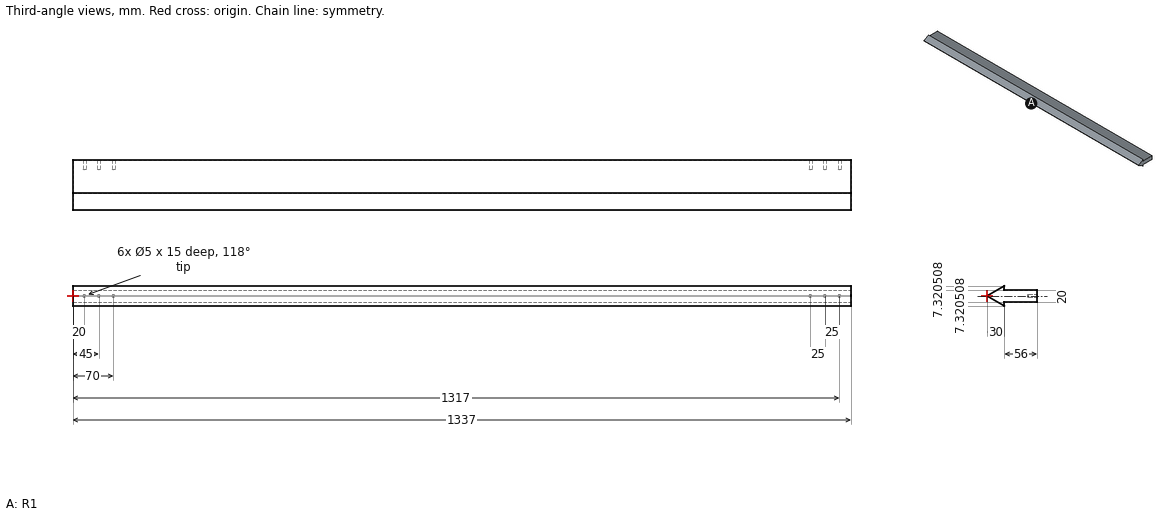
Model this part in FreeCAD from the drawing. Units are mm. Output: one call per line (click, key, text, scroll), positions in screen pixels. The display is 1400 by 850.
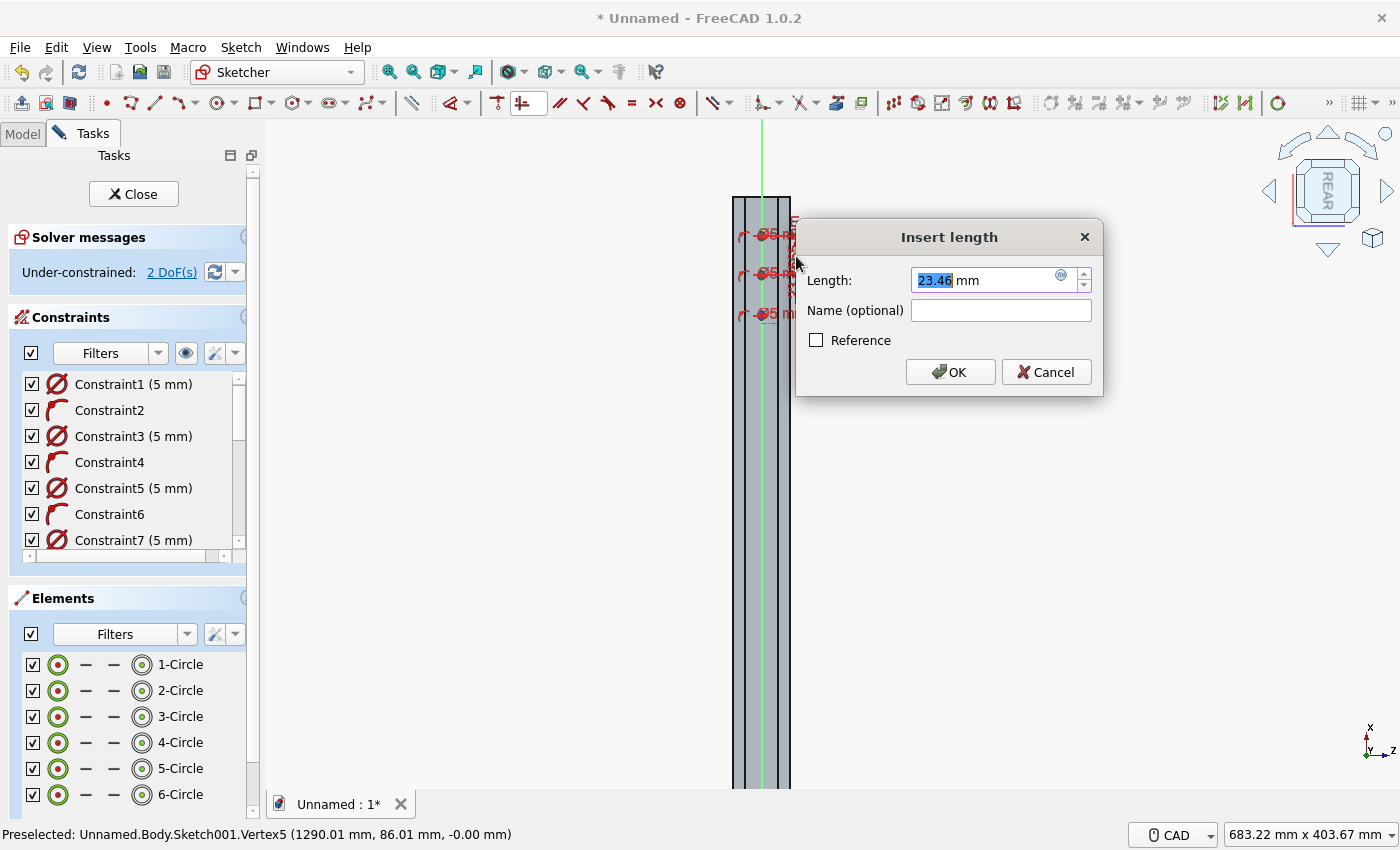
text(25)
key(Return)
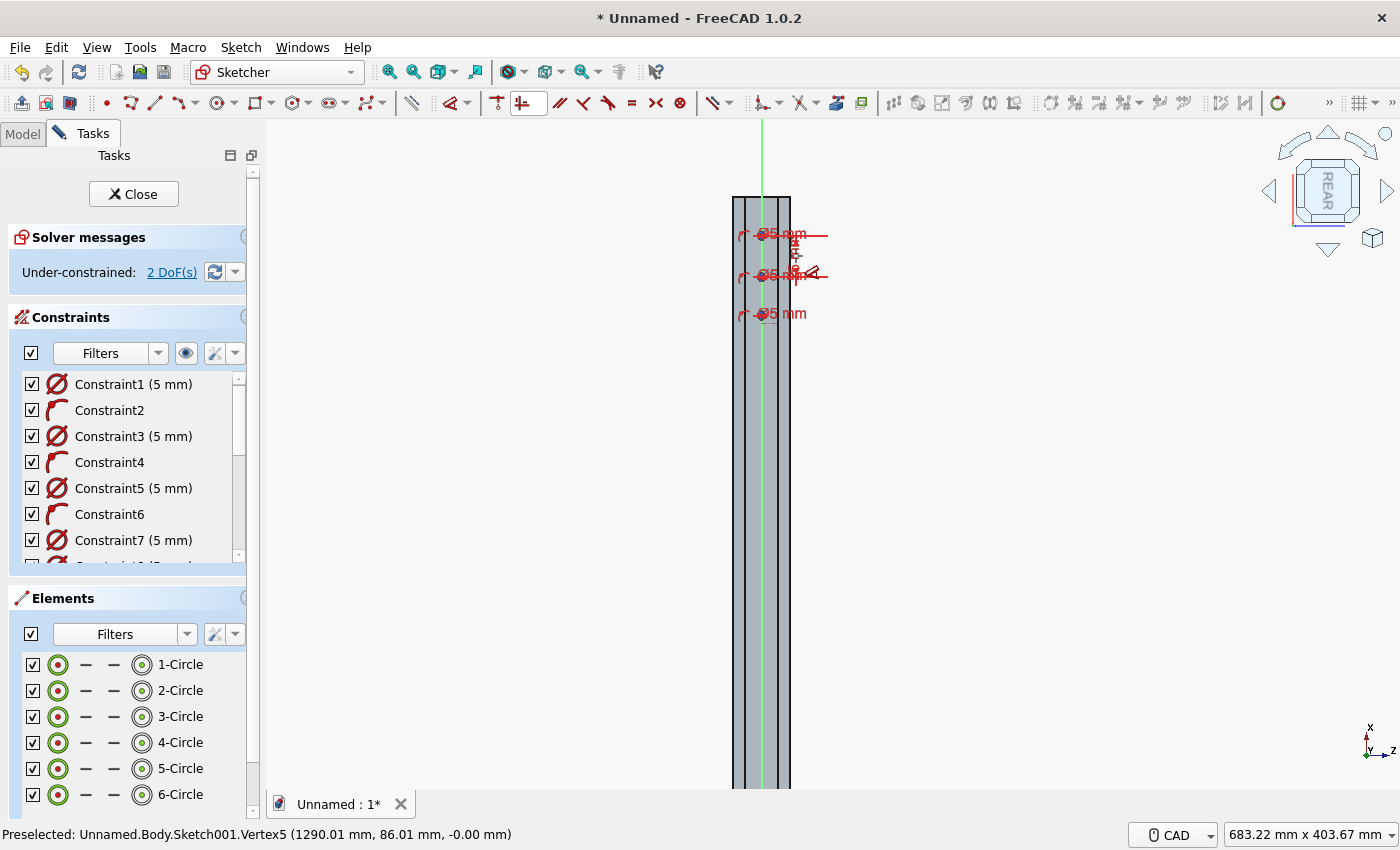
click(762, 277)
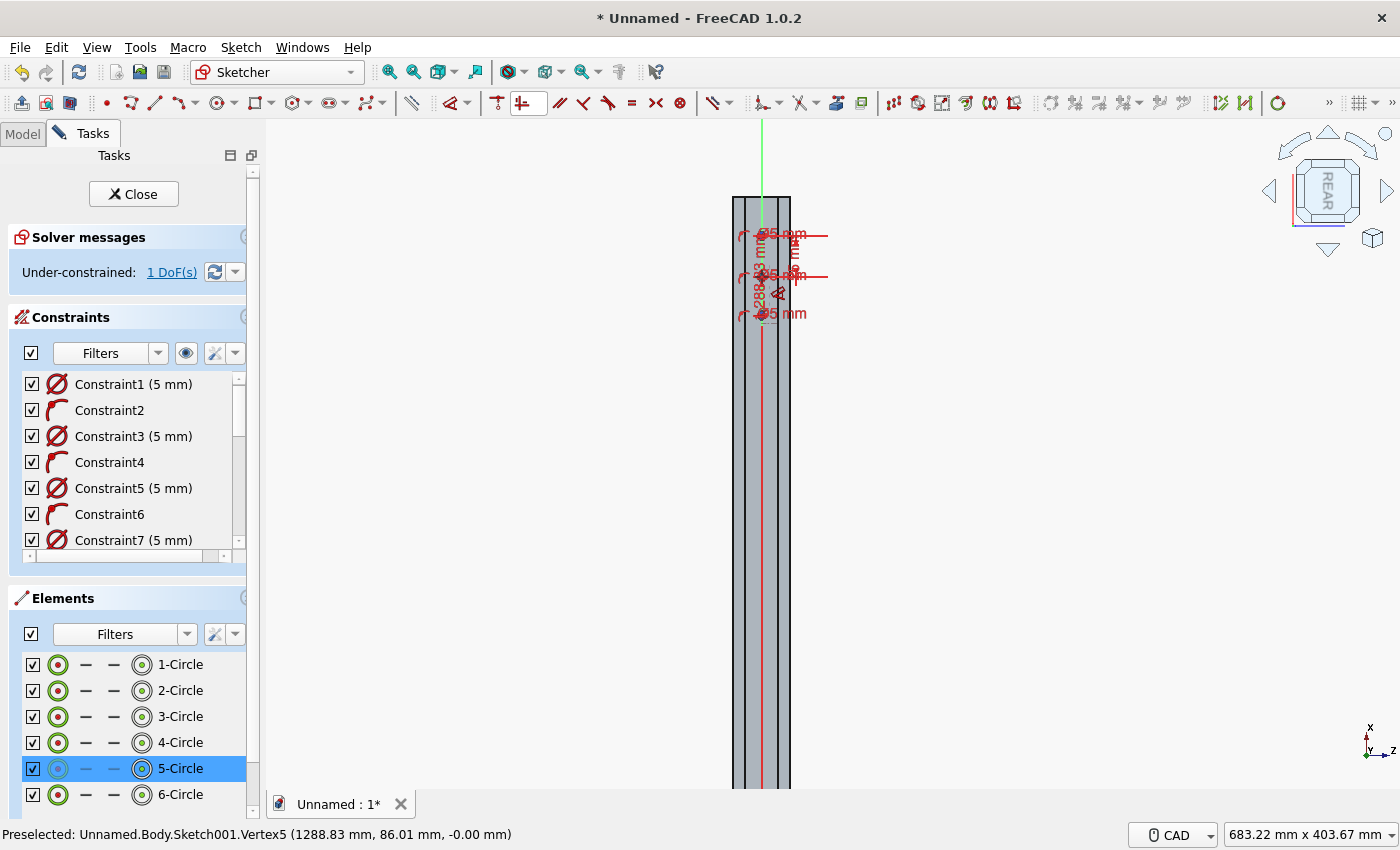
click(762, 316)
click(796, 296)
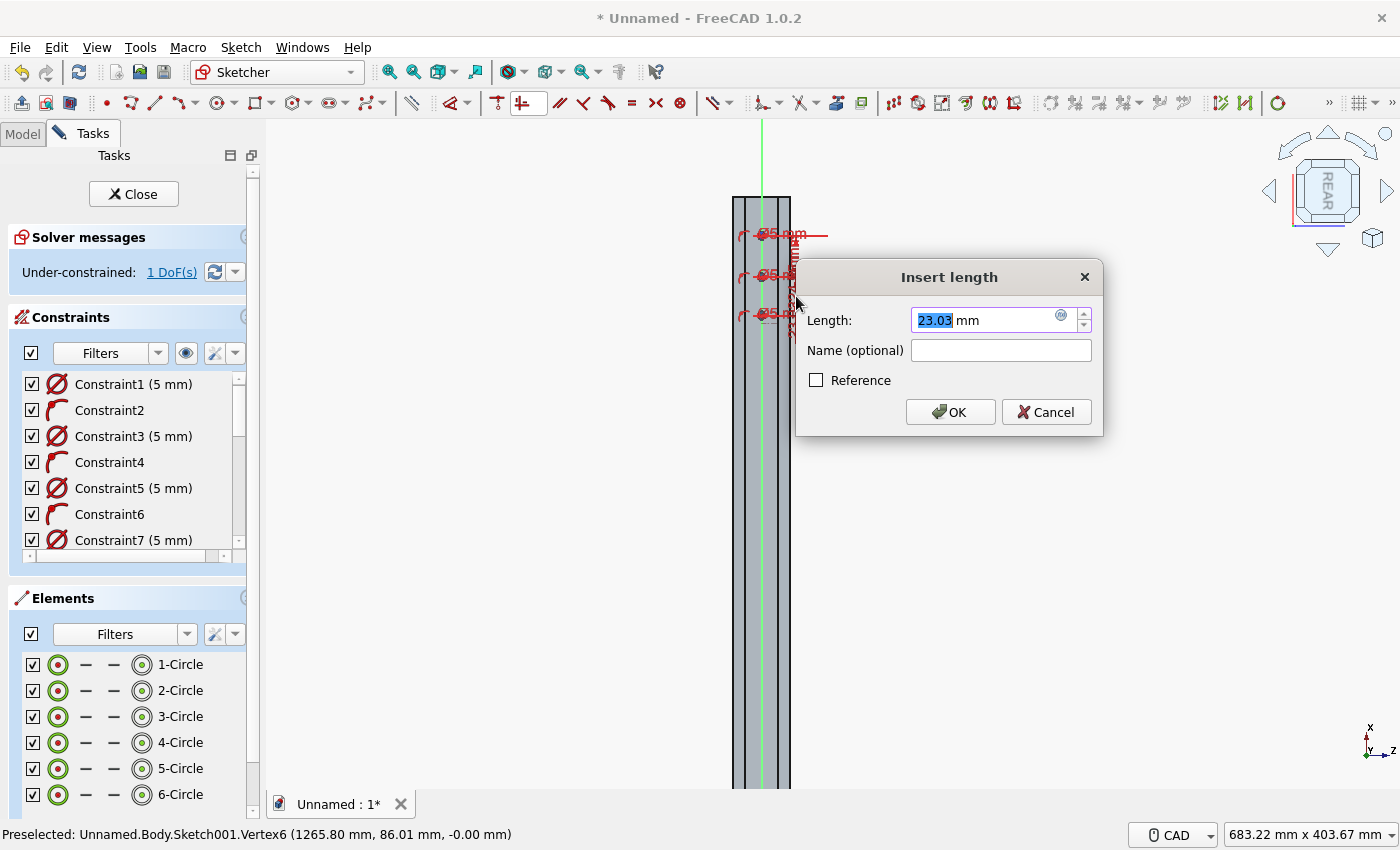
text(25)
key(Return)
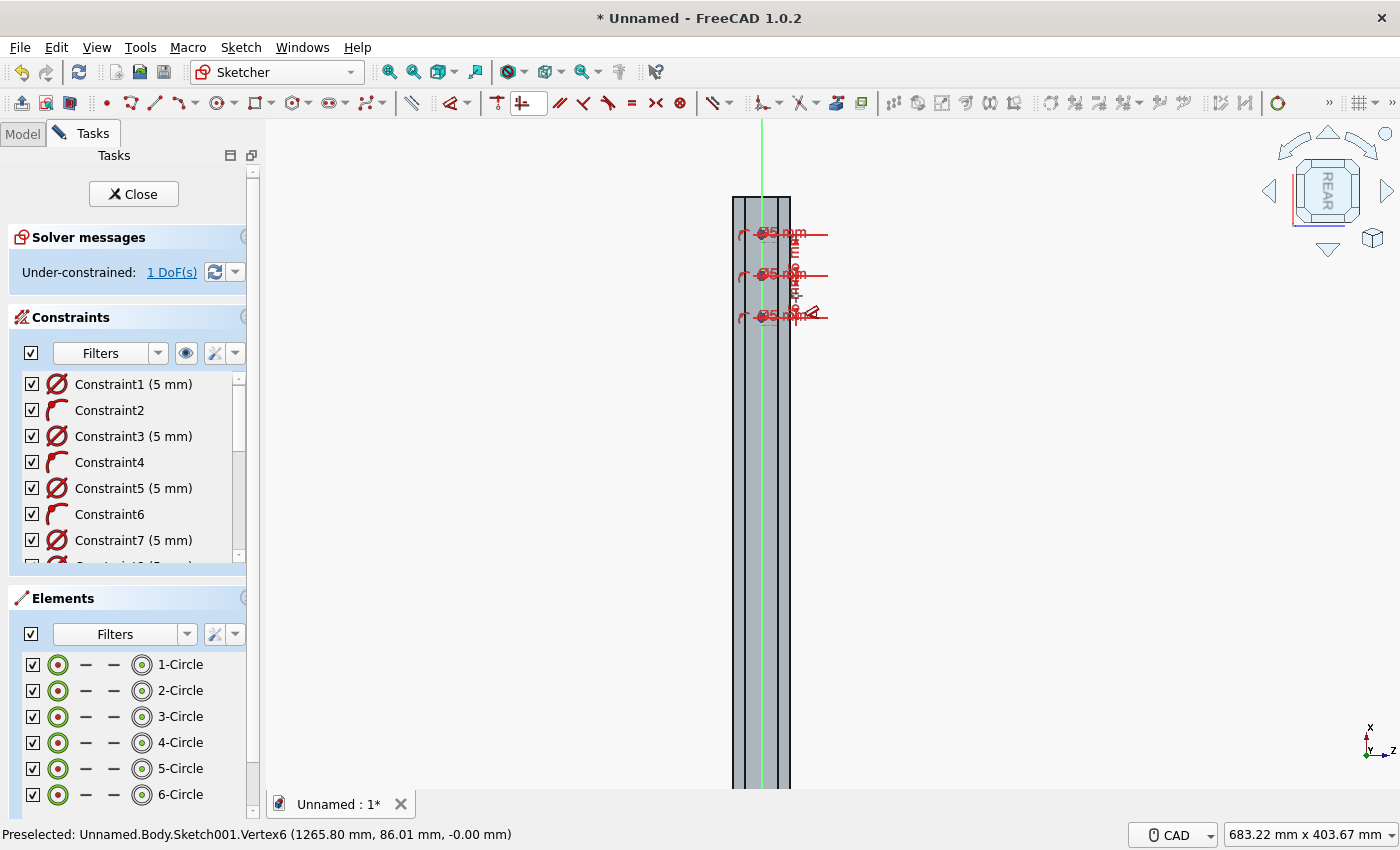
scroll(765, 235, down, 8)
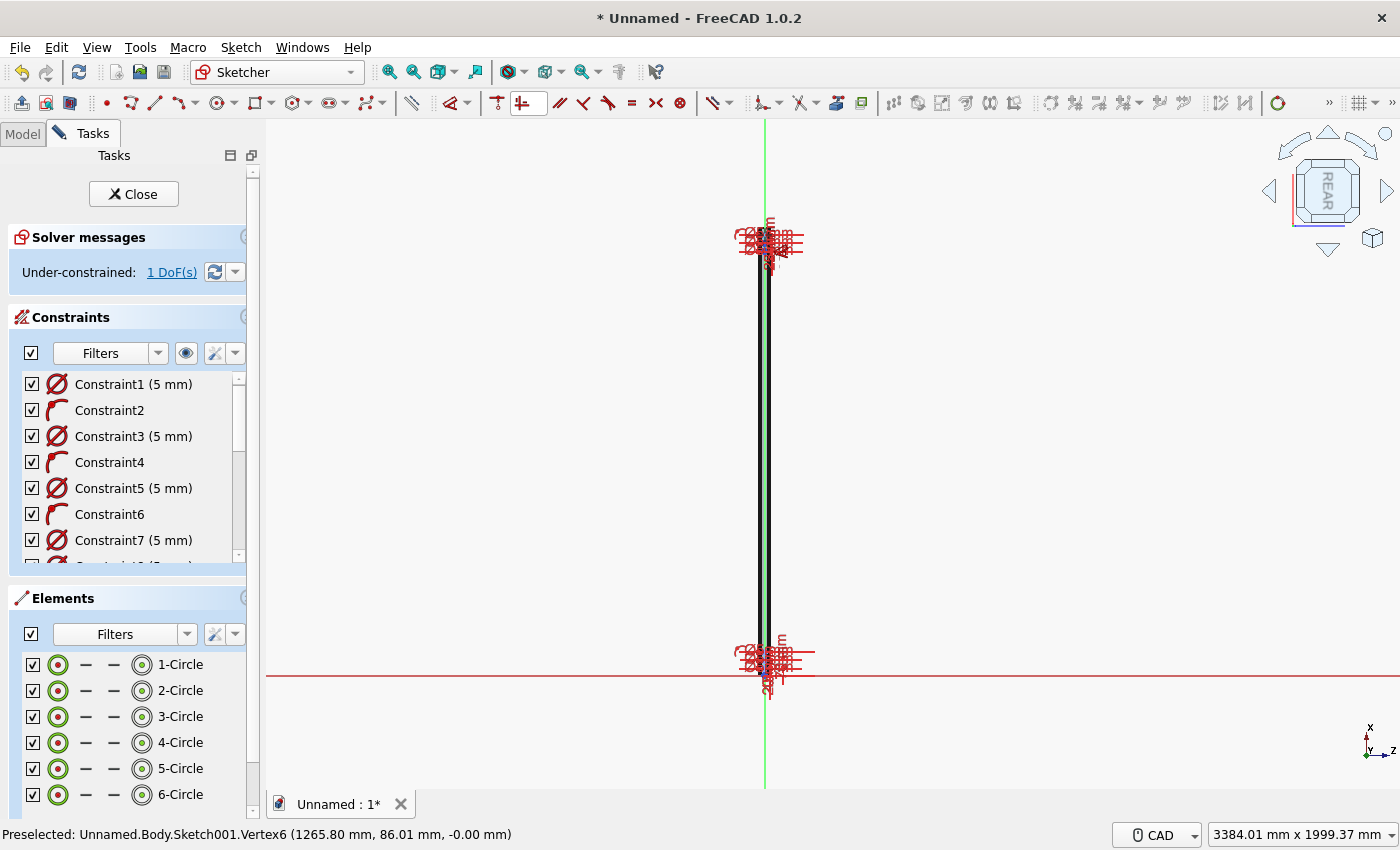
scroll(765, 235, up, 2)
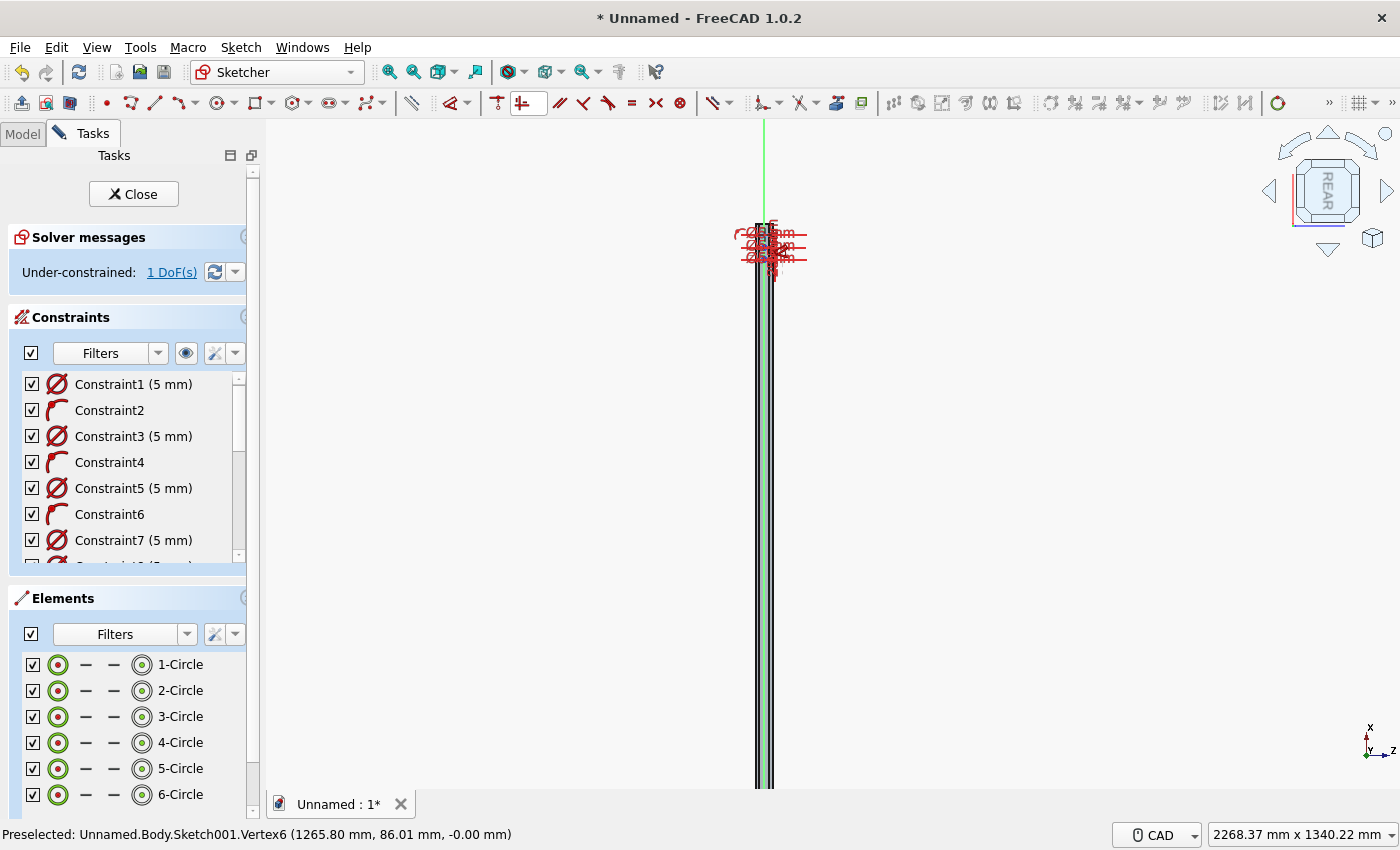
click(764, 235)
click(798, 498)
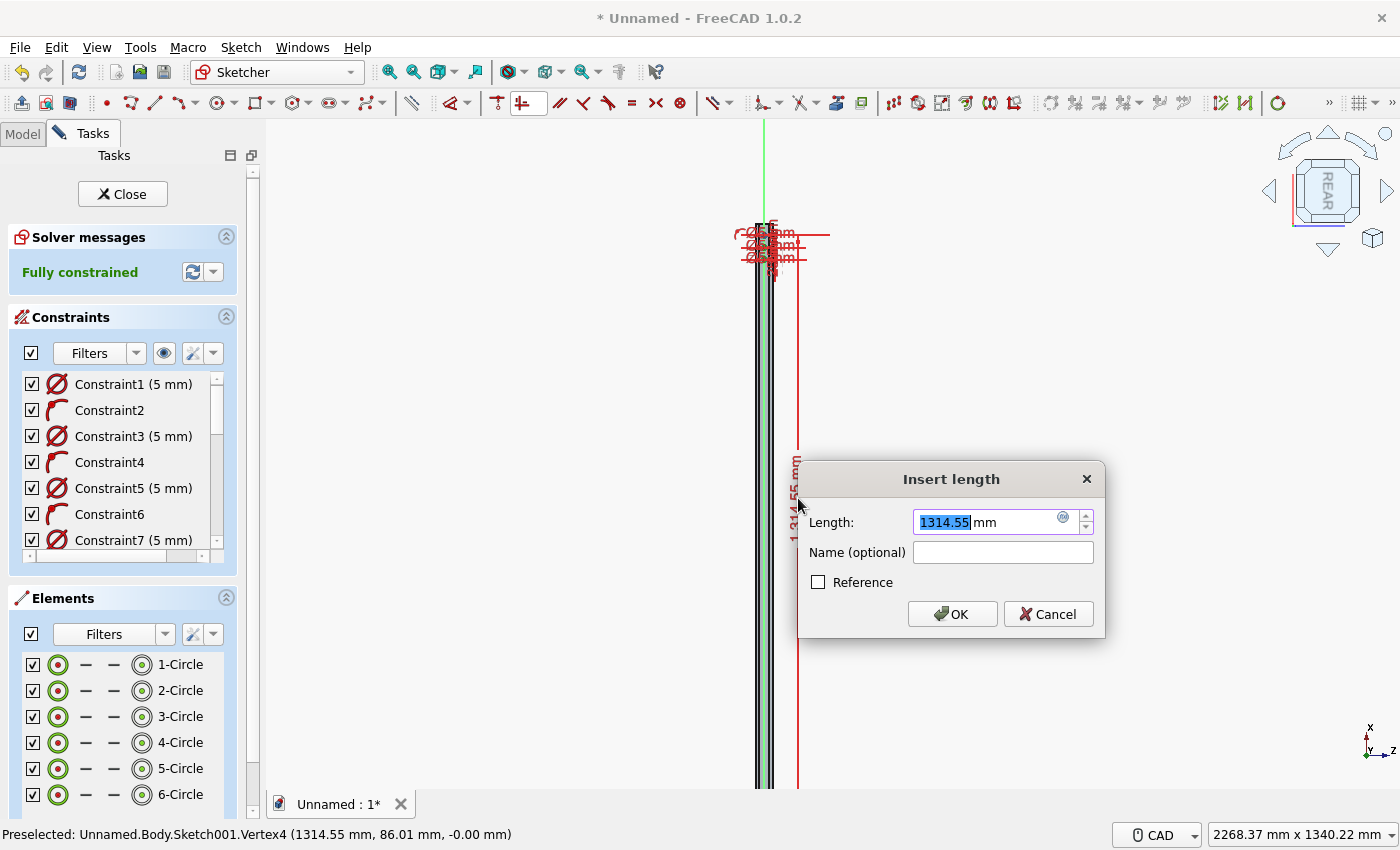
text(1317)
key(Return)
key(Escape)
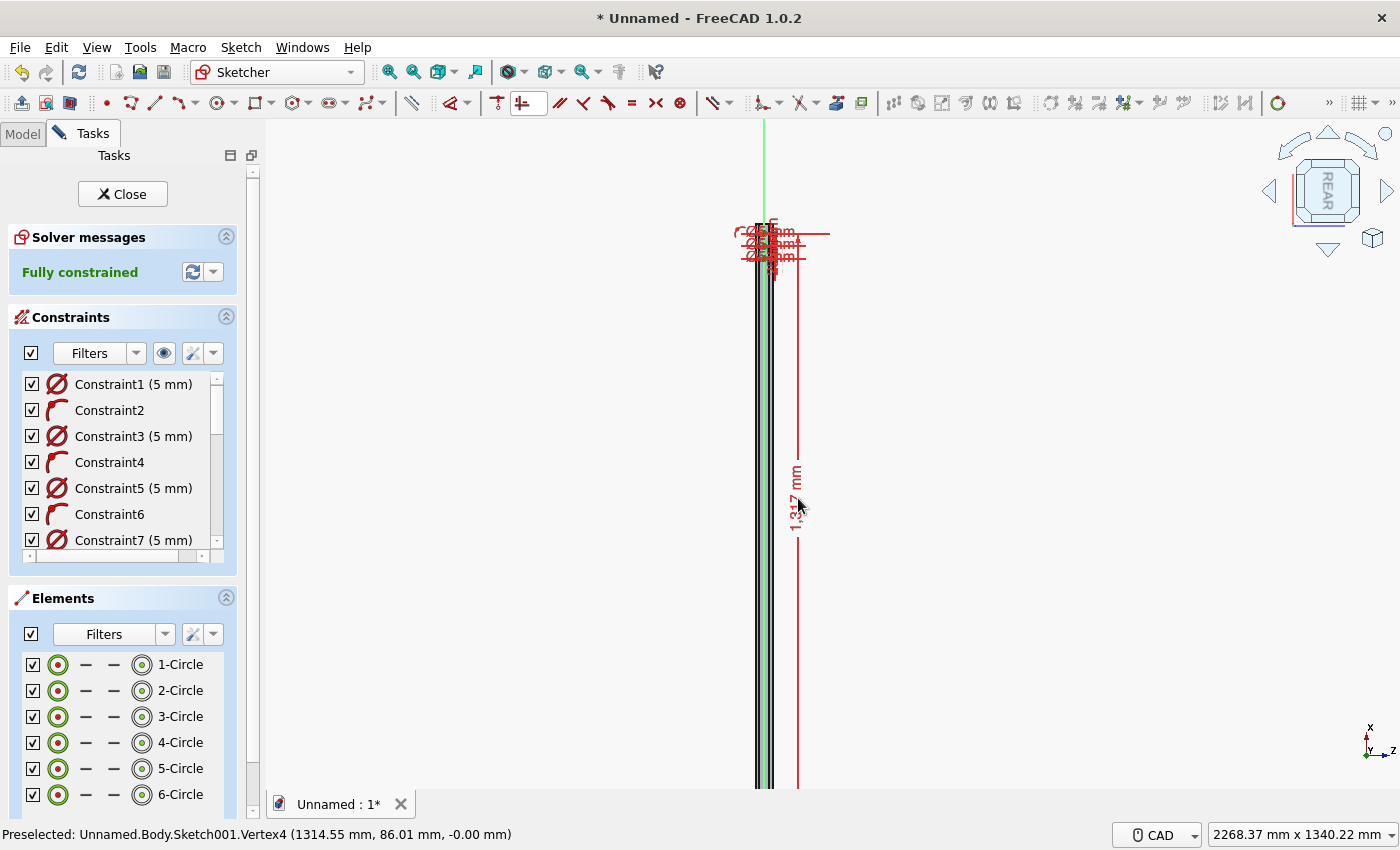
click(123, 194)